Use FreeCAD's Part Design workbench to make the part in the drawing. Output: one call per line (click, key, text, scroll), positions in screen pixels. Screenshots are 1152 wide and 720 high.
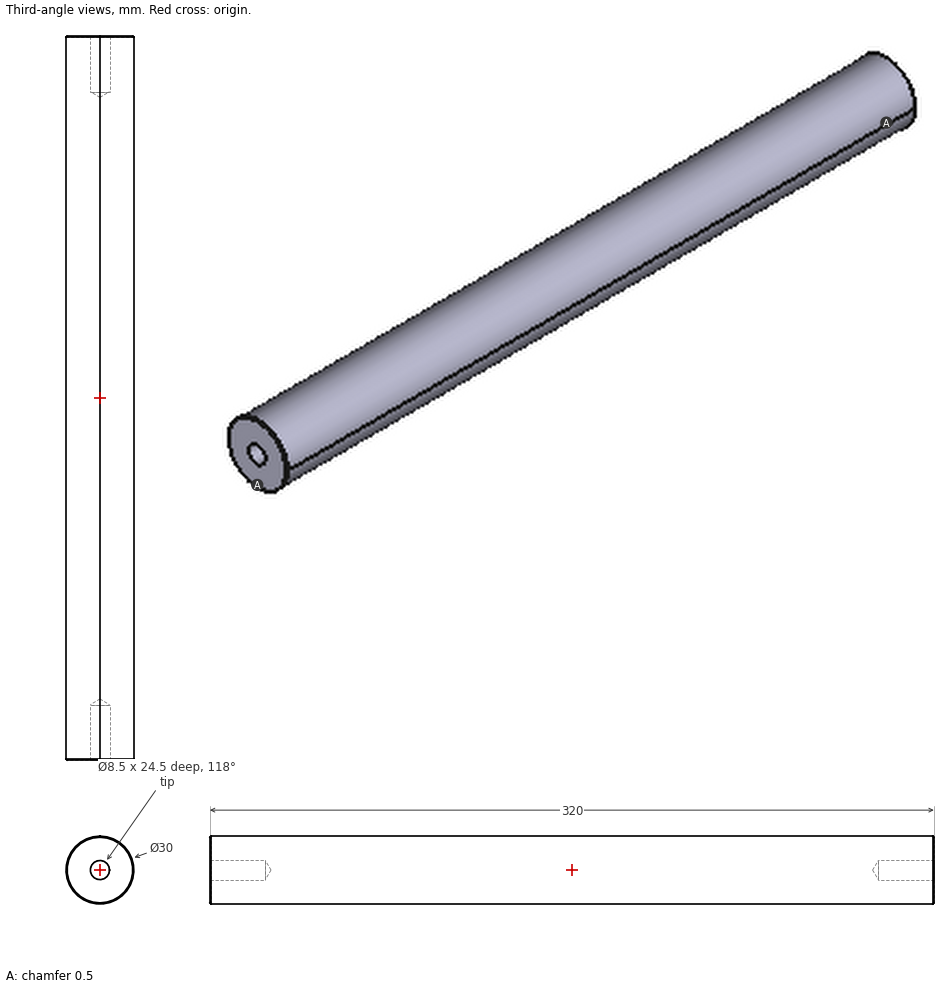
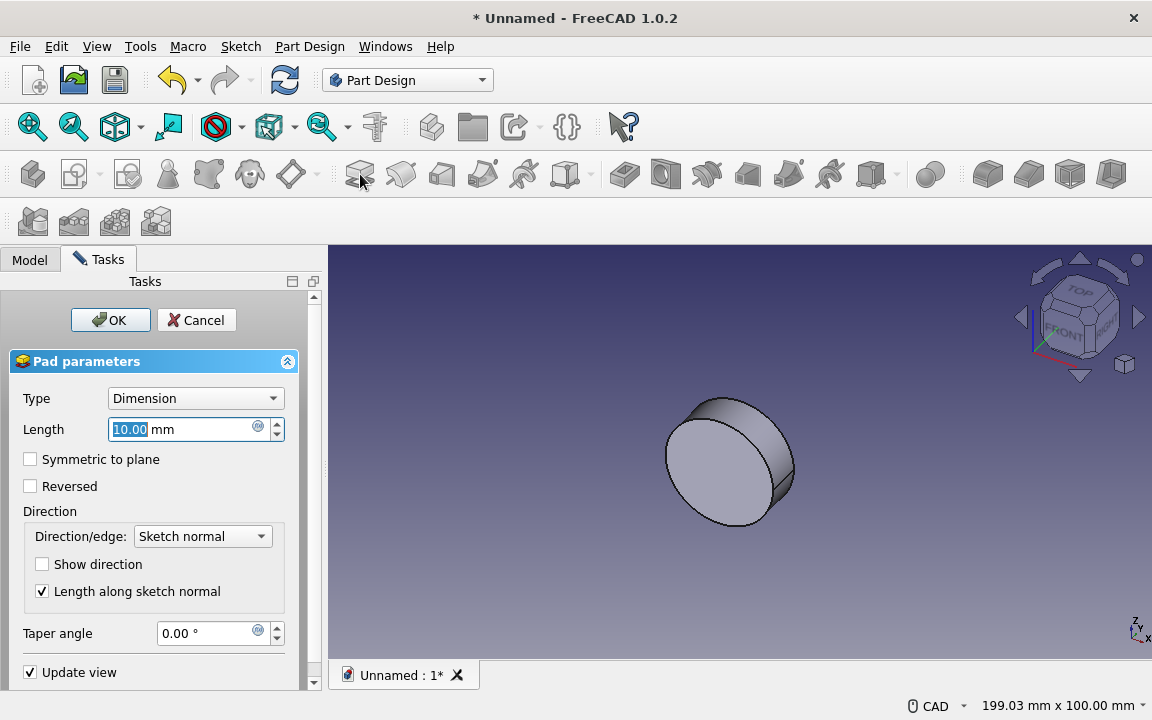
text(320)
key(Tab)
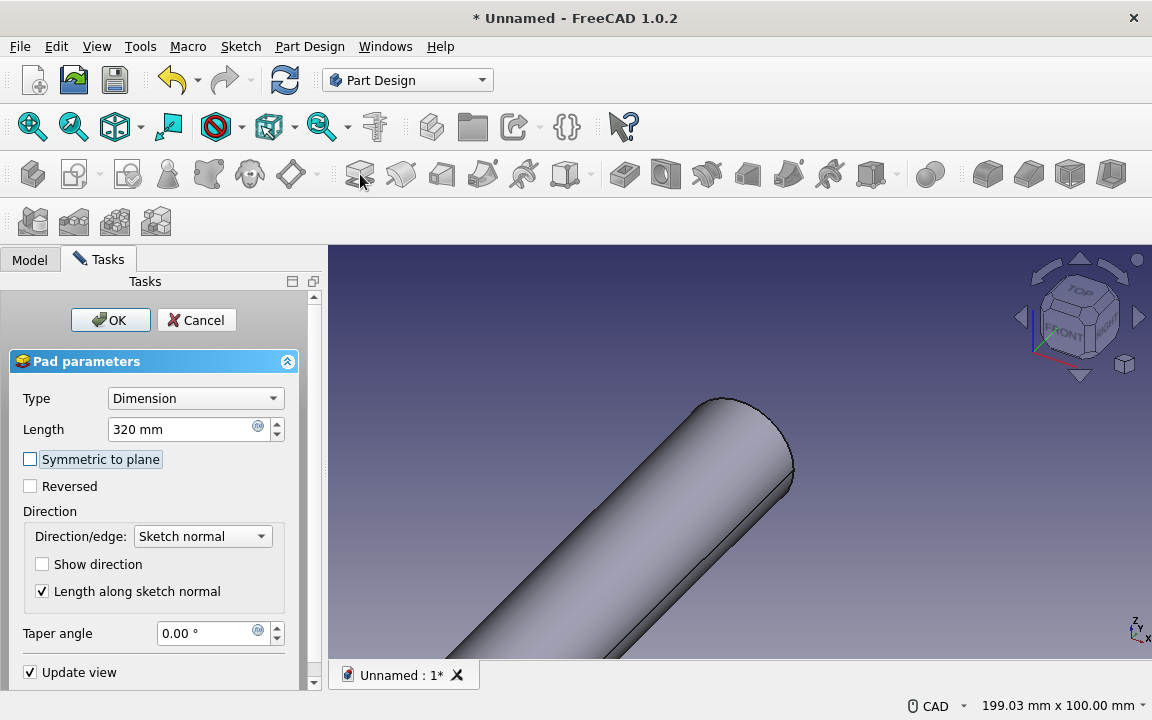
click(31, 459)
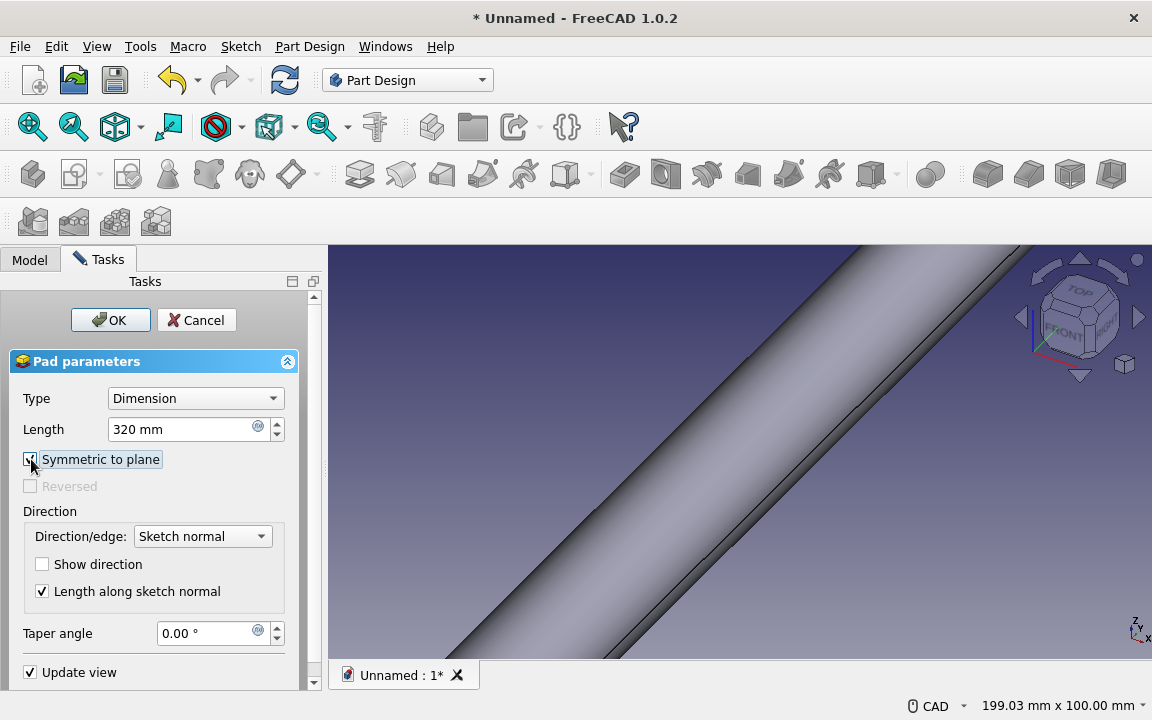
click(111, 320)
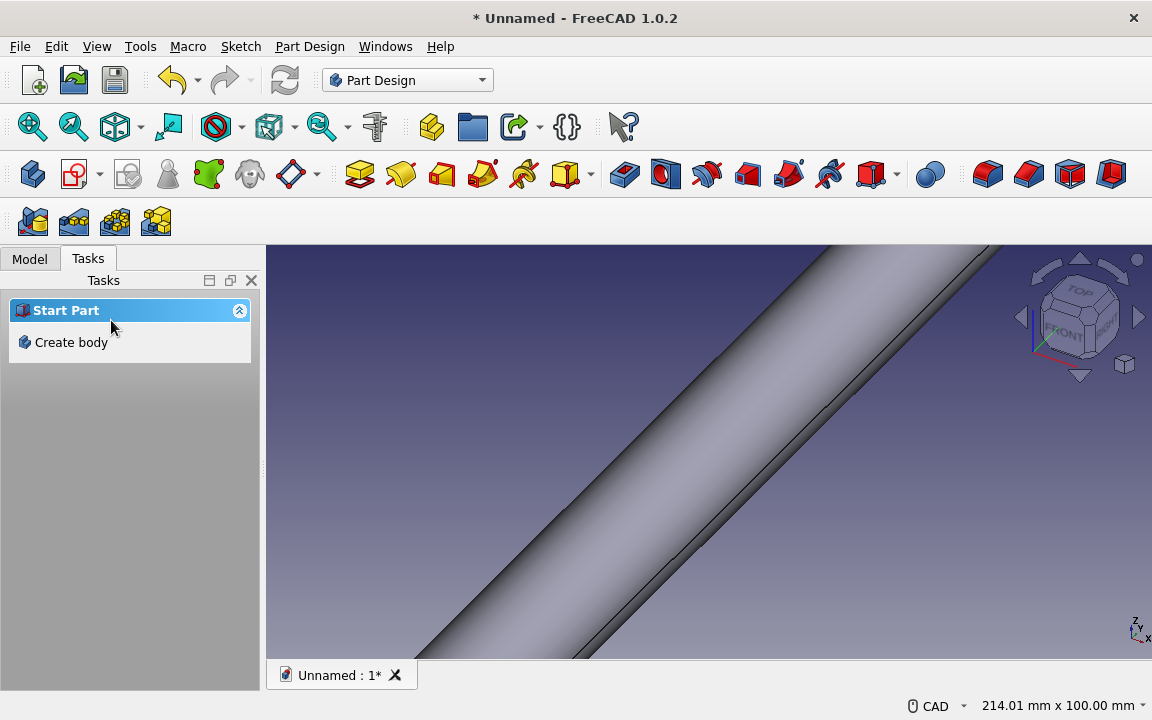
key(v)
key(f)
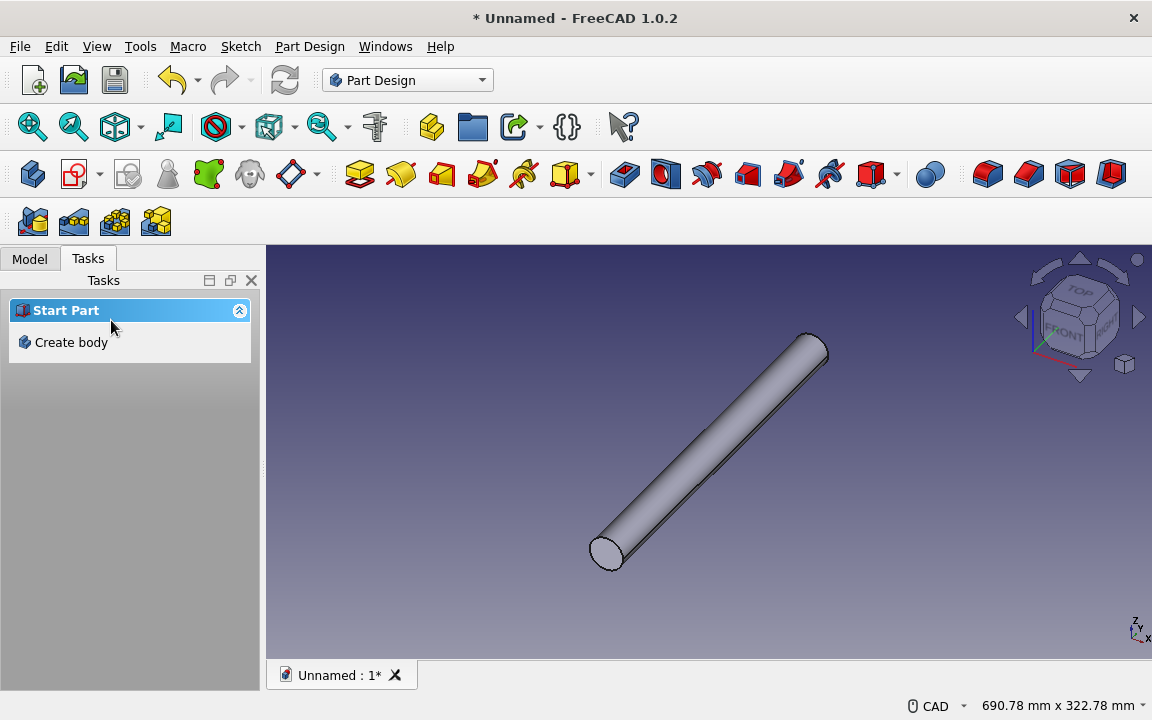
click(593, 539)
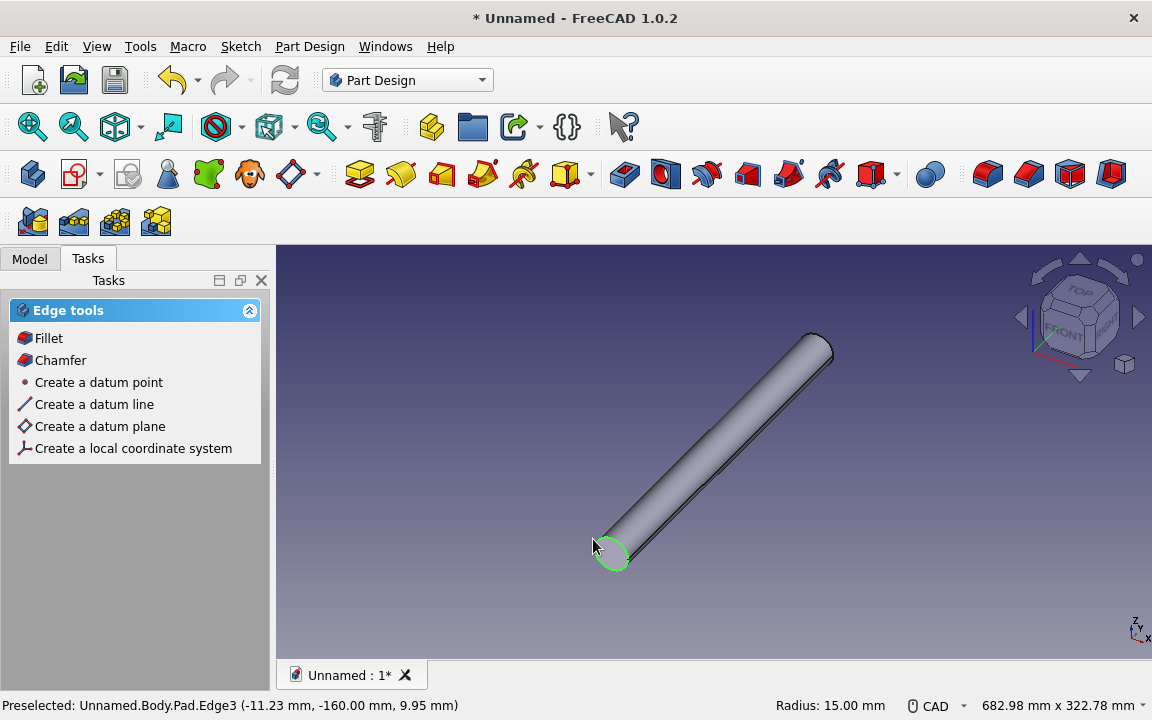
click(811, 332, ctrl)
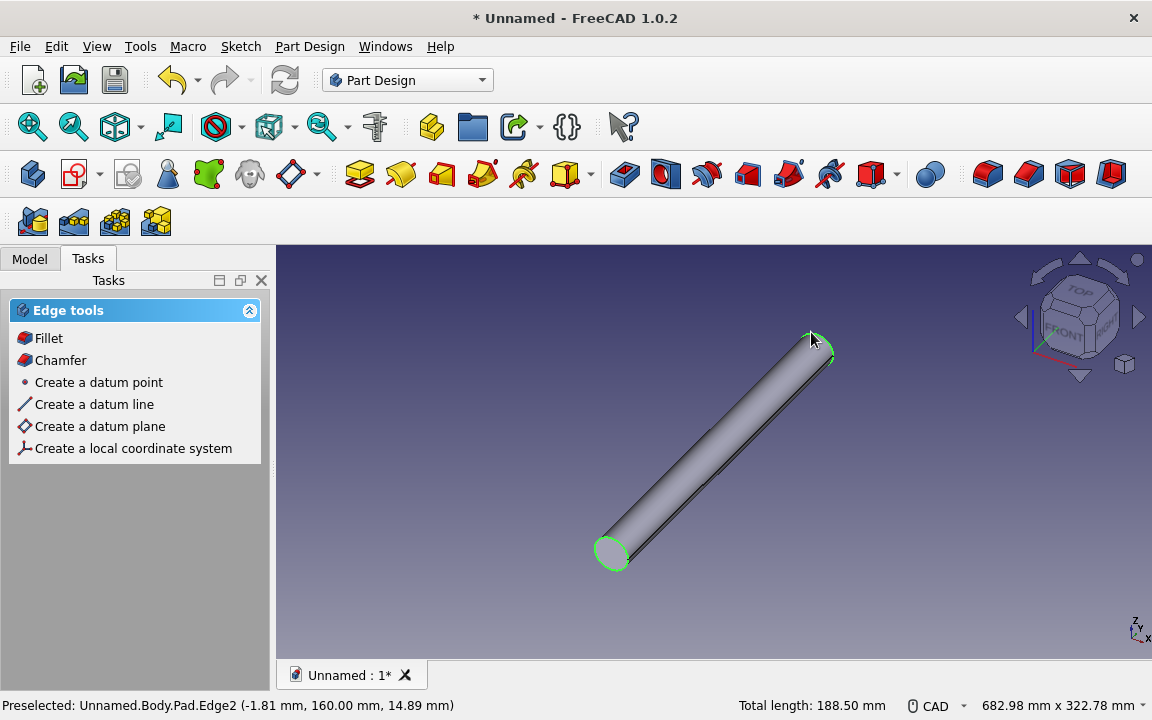
click(1029, 174)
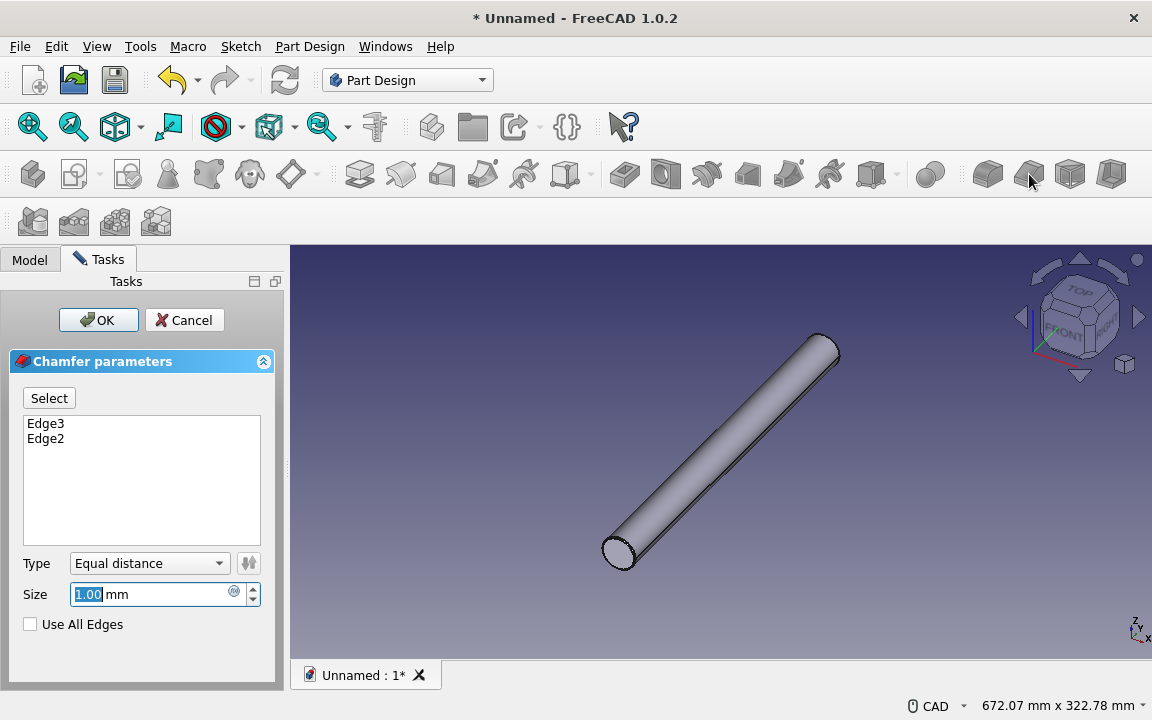
text(0.5)
key(Tab)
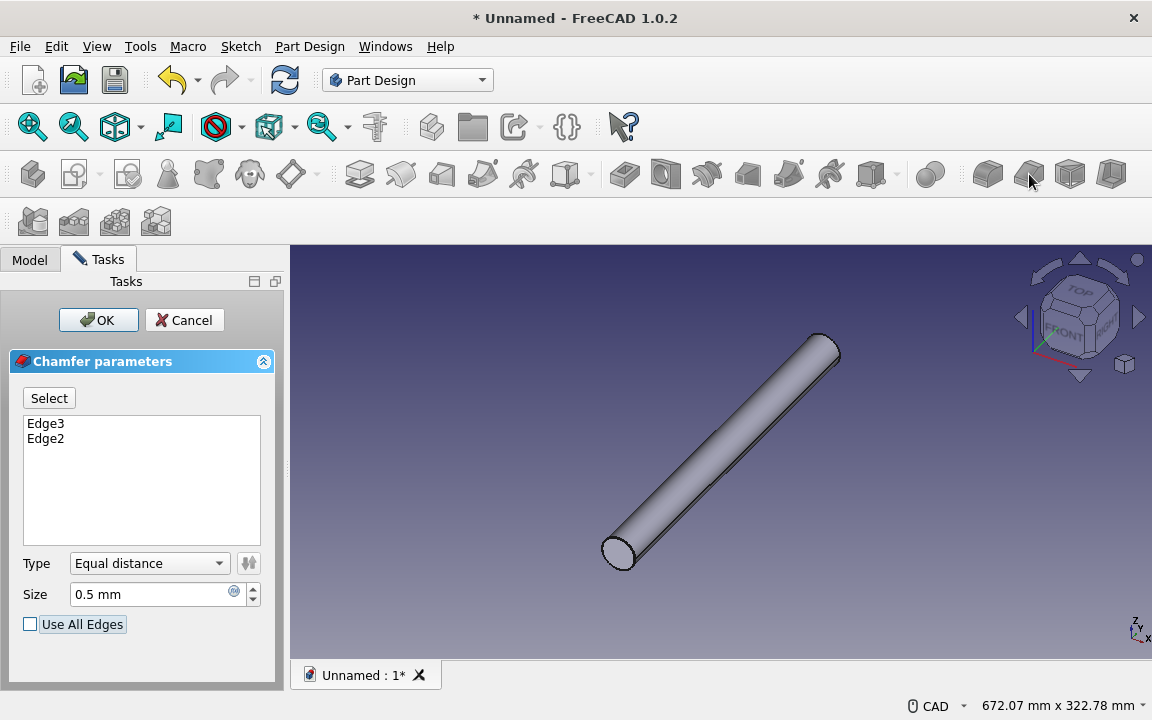
click(99, 320)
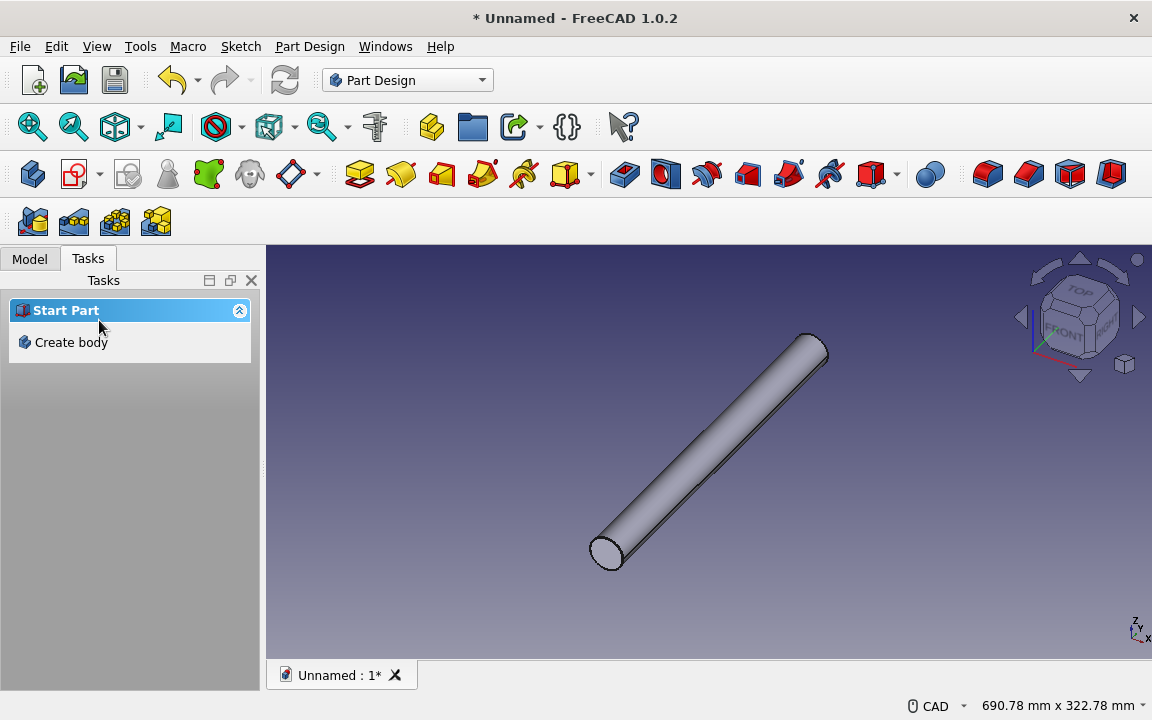
key(4)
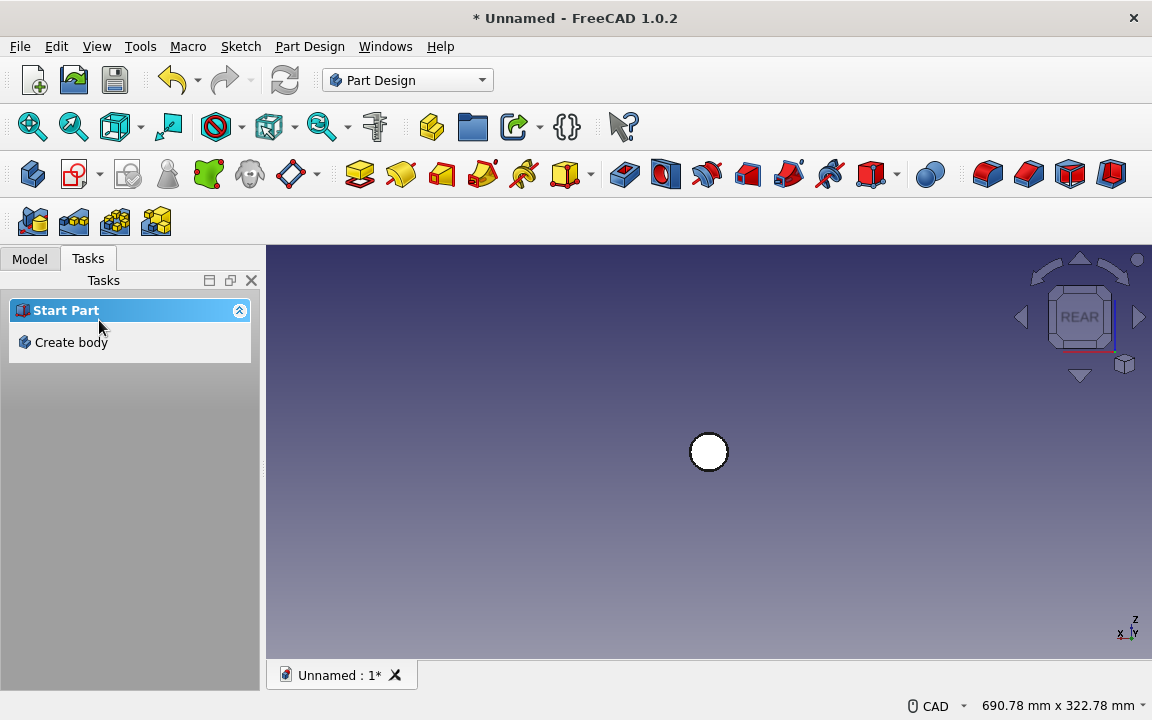
key(v)
key(f)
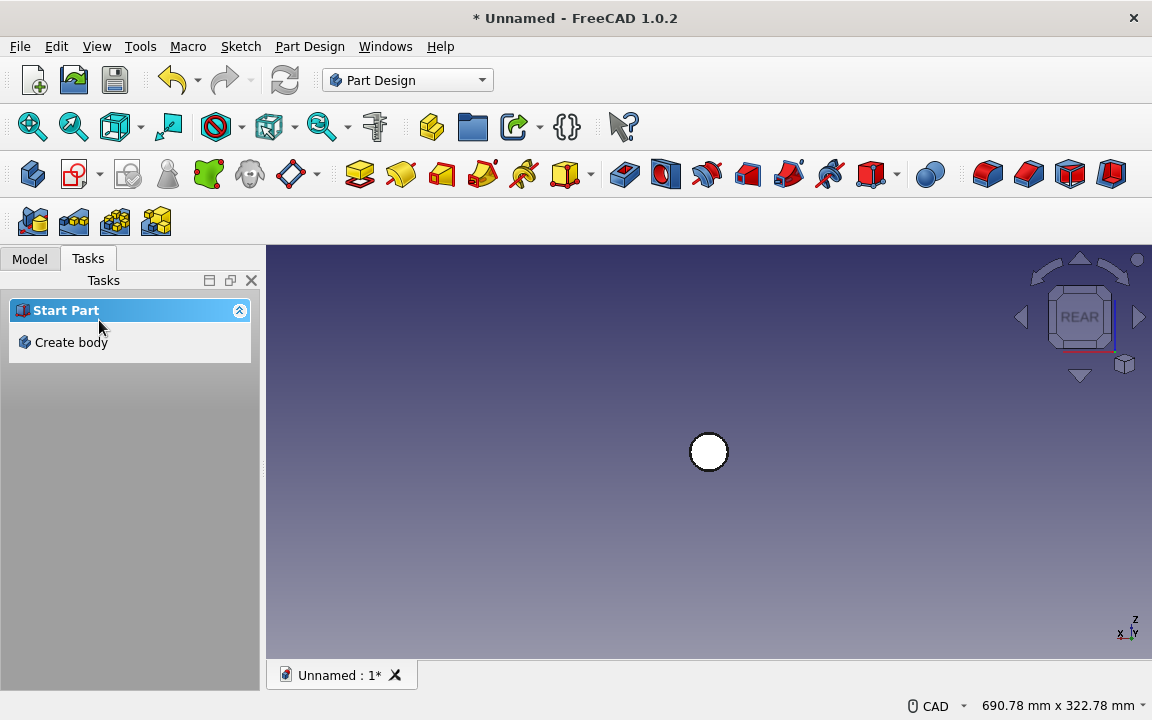
click(709, 451)